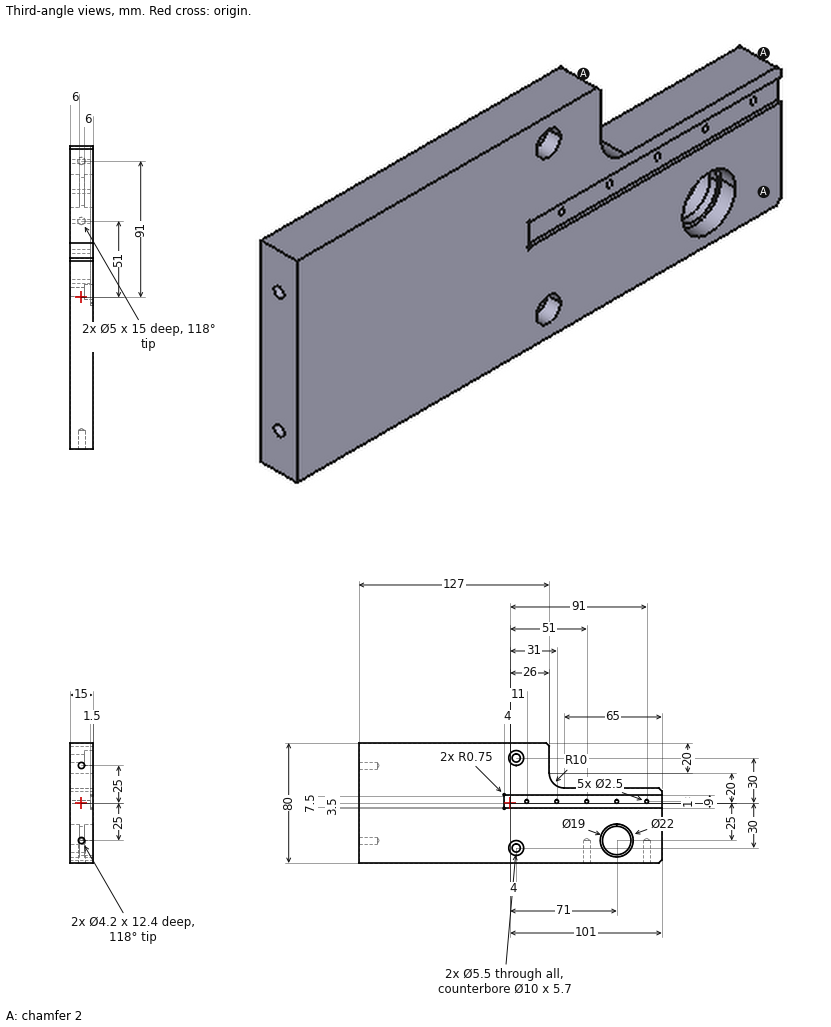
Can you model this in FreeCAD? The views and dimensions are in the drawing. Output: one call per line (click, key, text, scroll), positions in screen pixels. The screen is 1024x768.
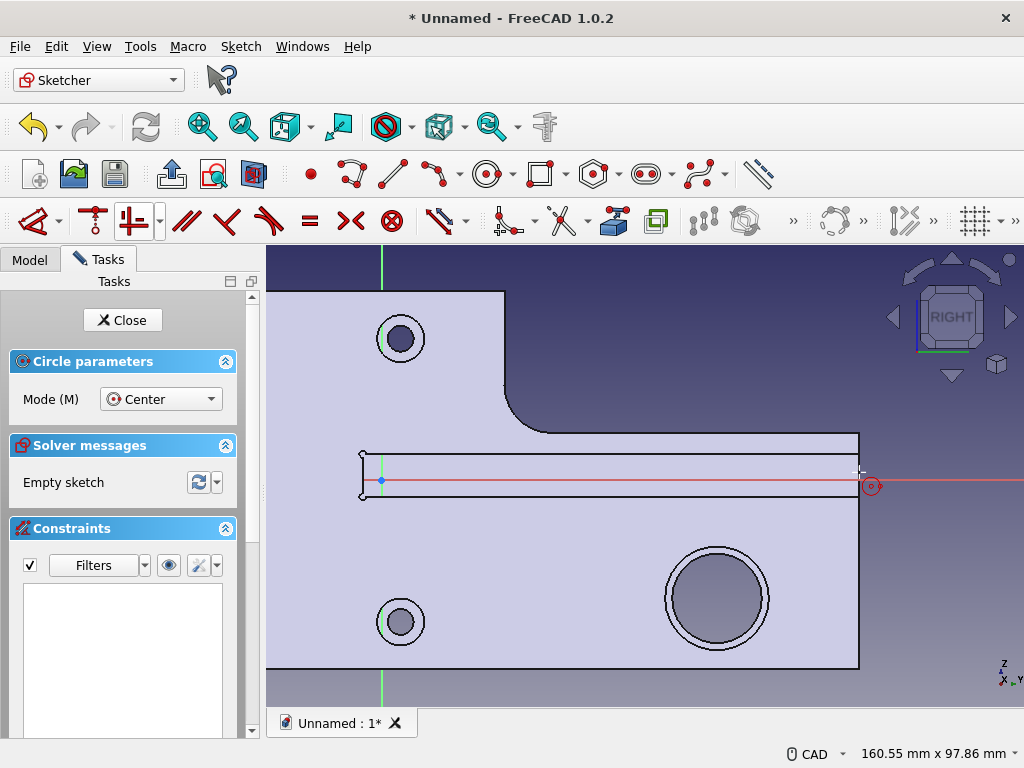
scroll(811, 476, up, 7)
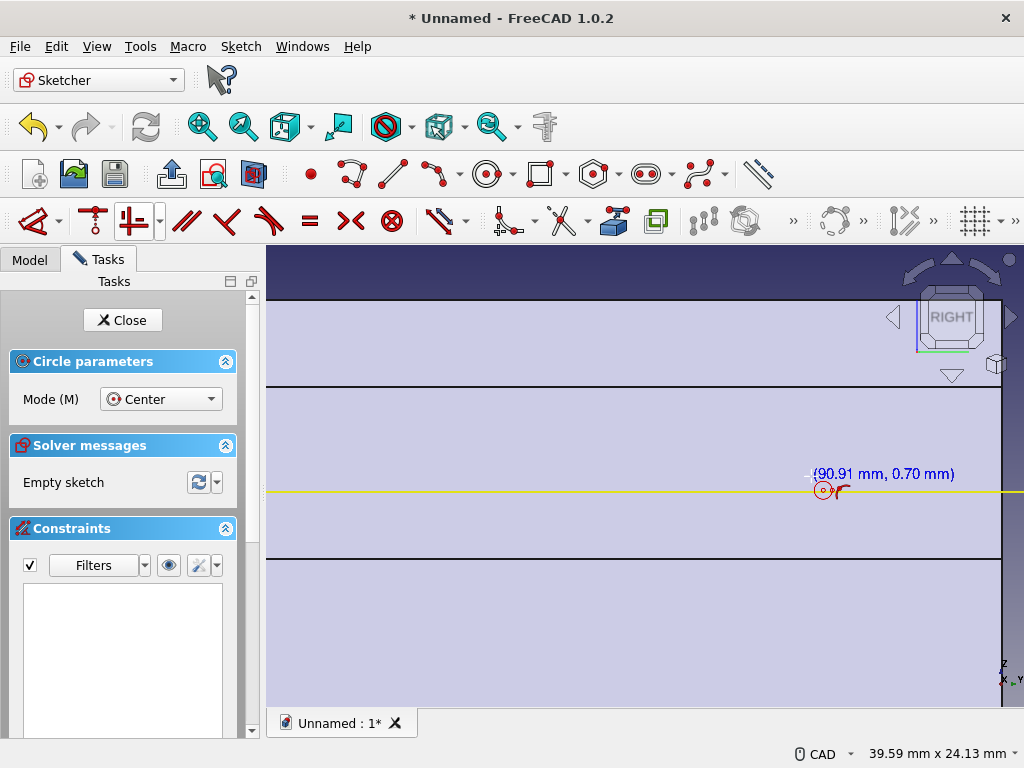
click(810, 473)
click(827, 456)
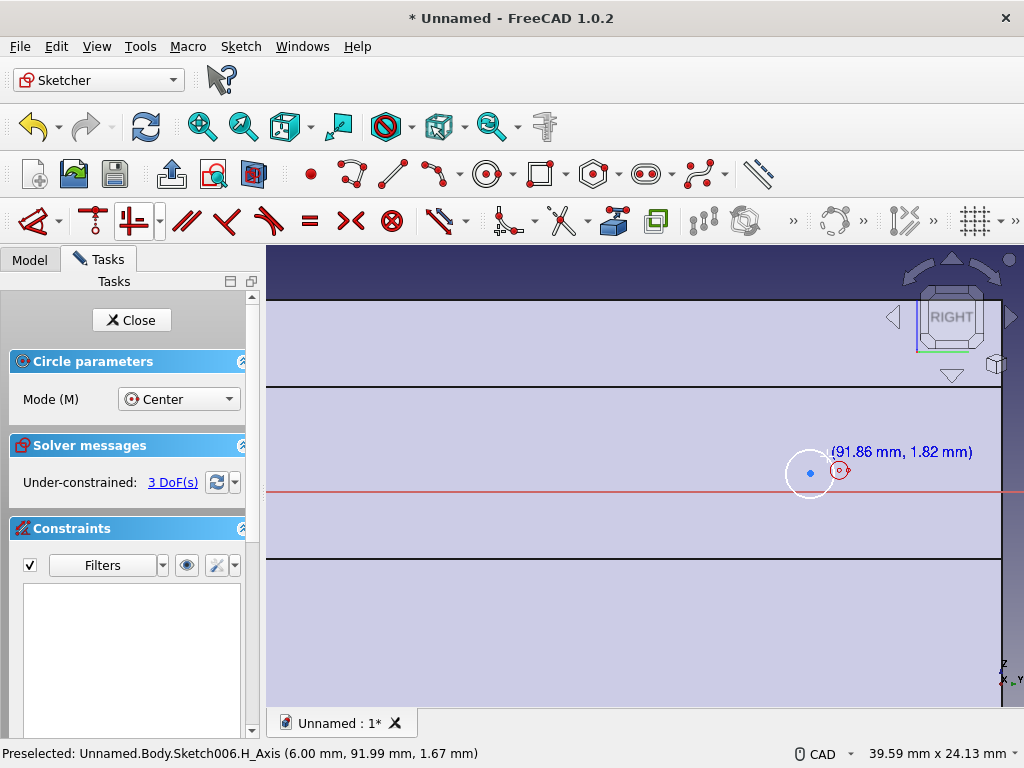
click(428, 473)
click(444, 456)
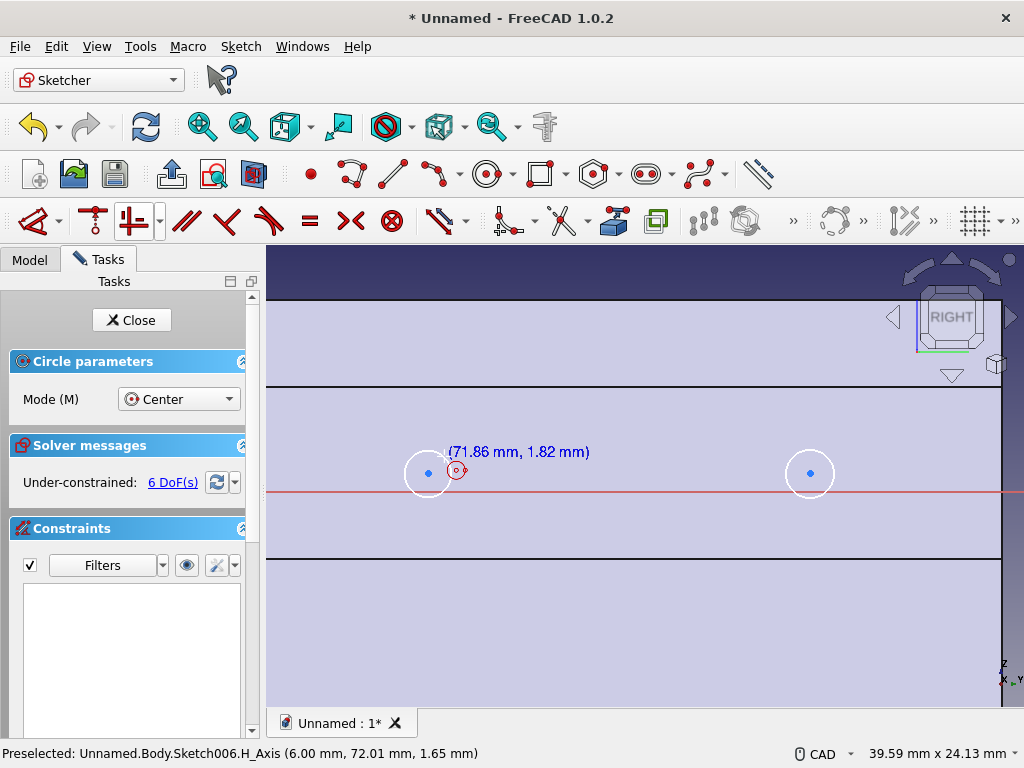
scroll(781, 477, down, 7)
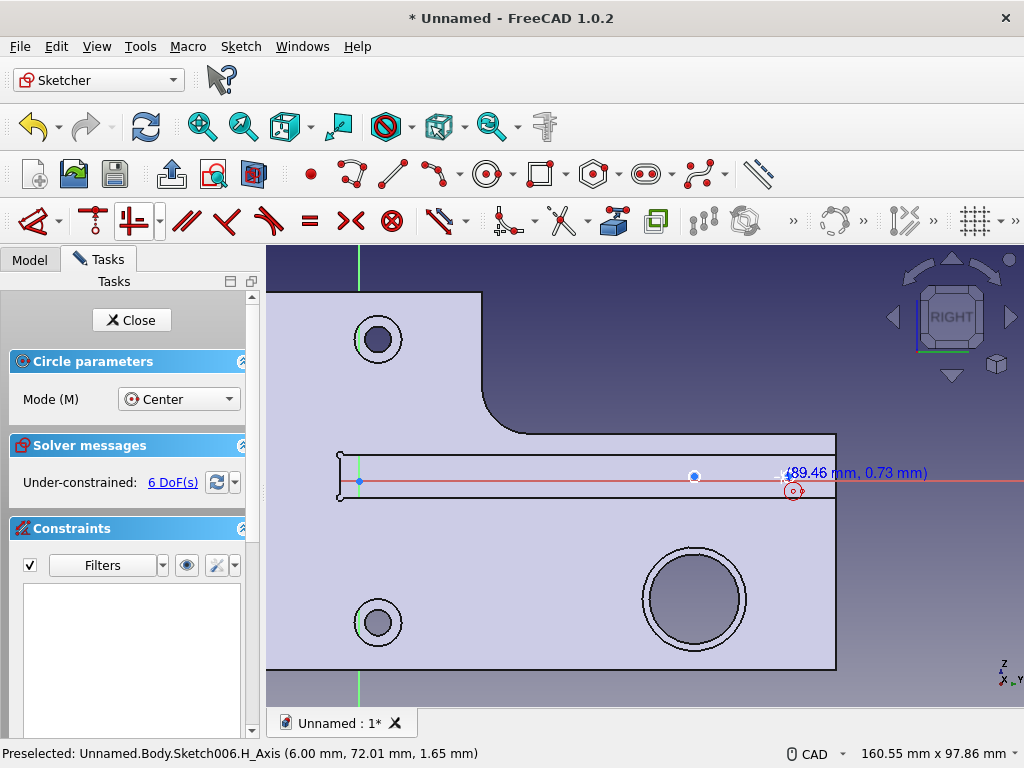
scroll(600, 476, up, 7)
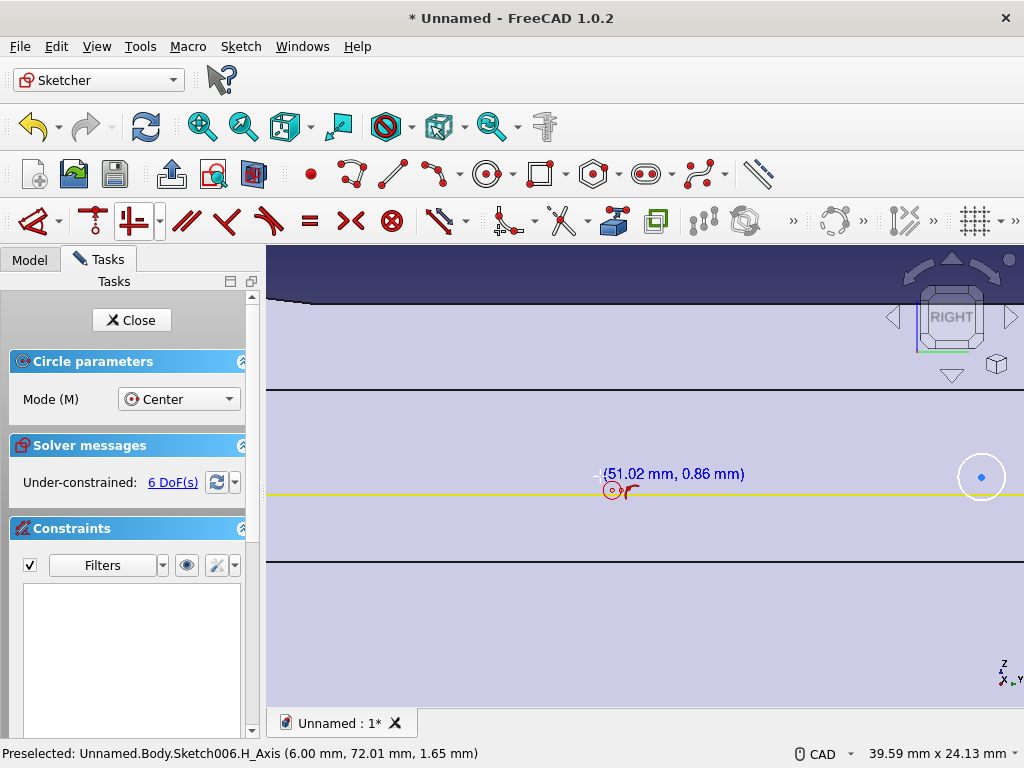
click(598, 476)
click(615, 459)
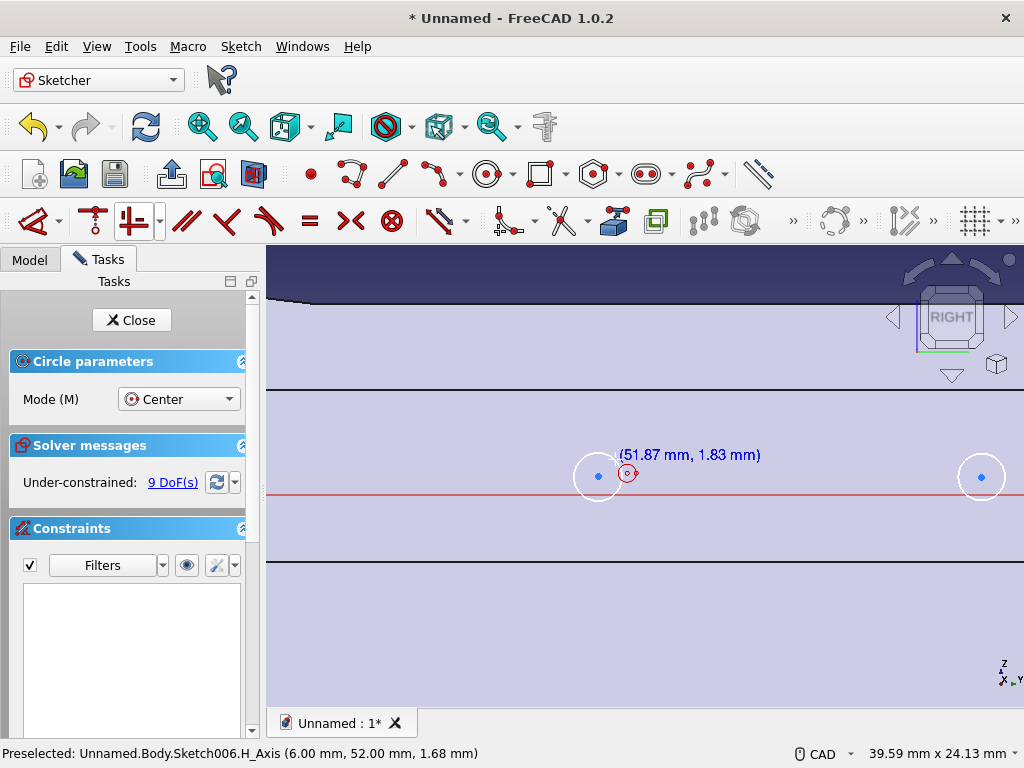
scroll(600, 476, down, 7)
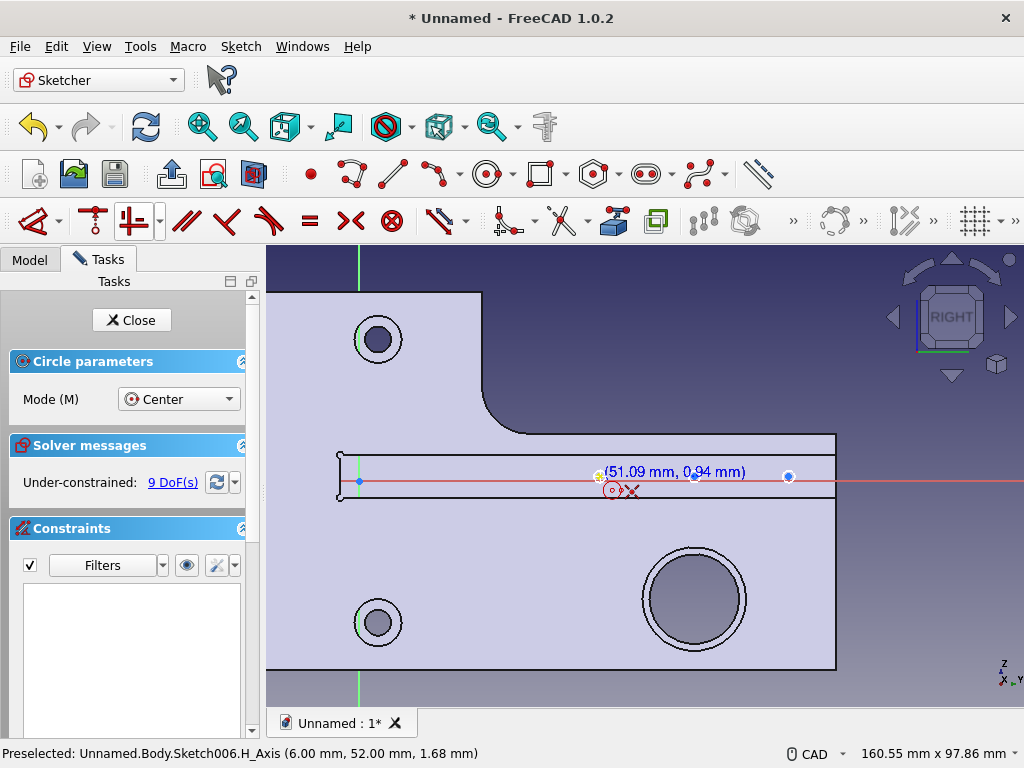
scroll(506, 476, up, 7)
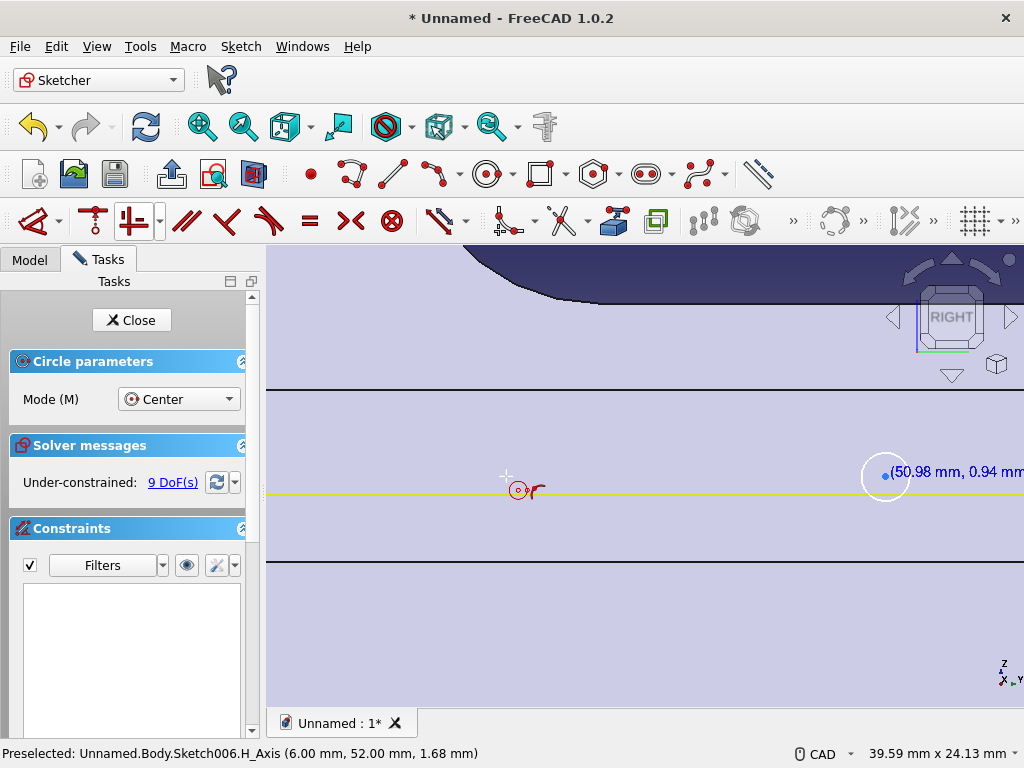
click(503, 476)
click(520, 459)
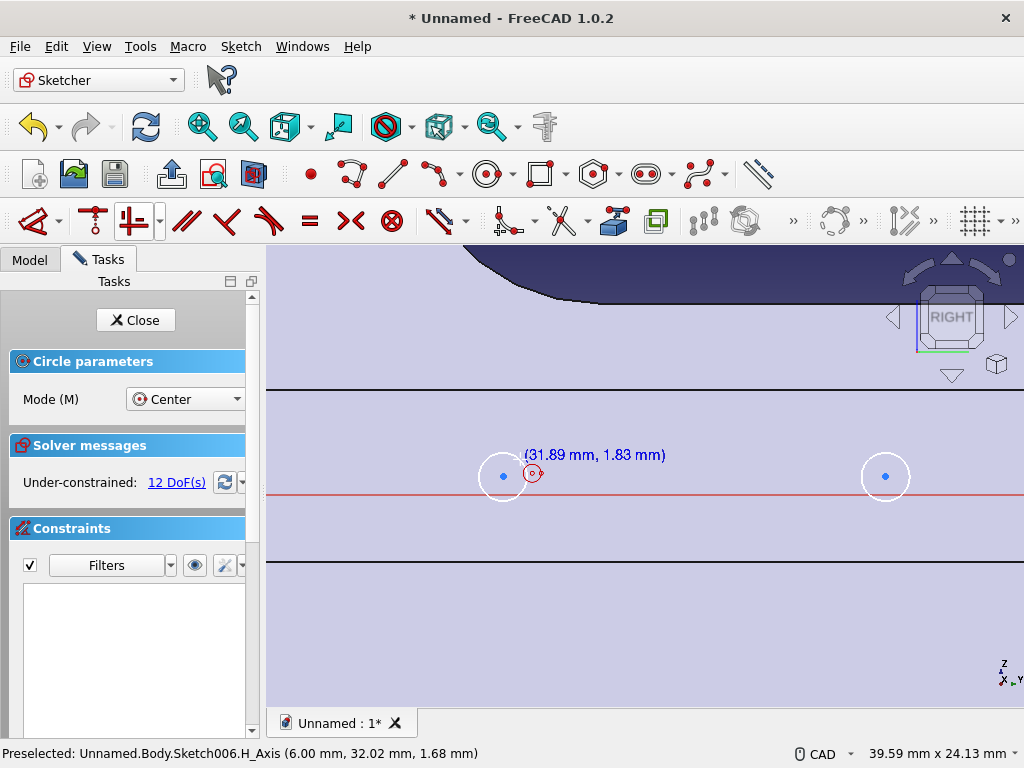
scroll(506, 476, down, 7)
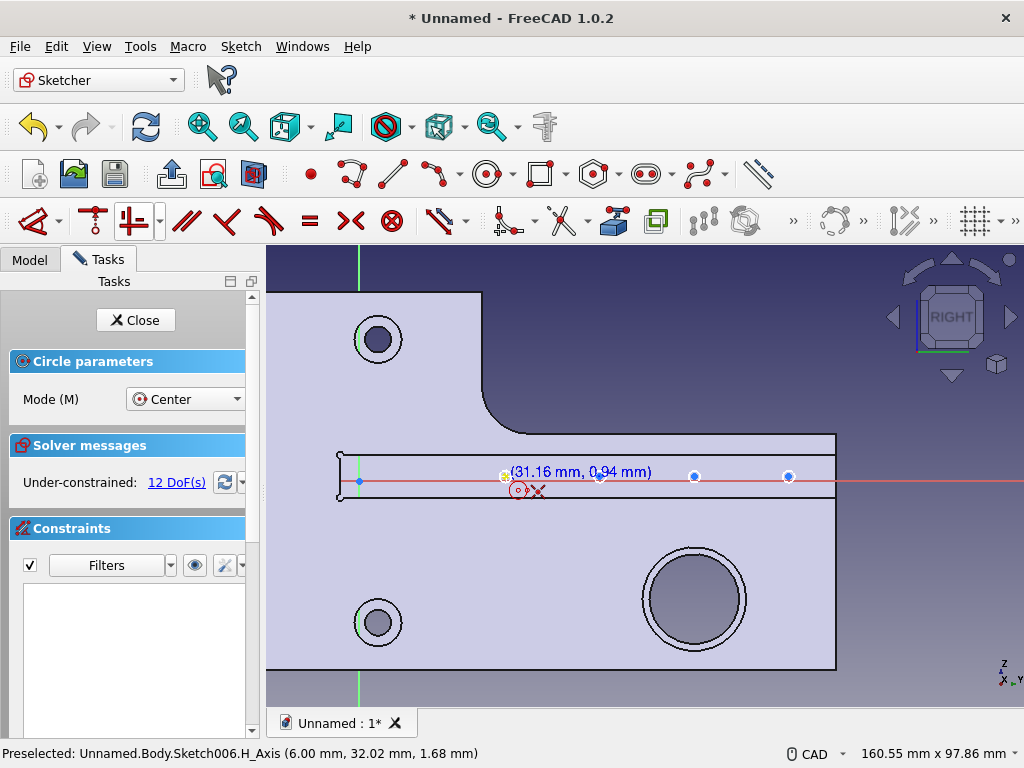
scroll(411, 476, up, 7)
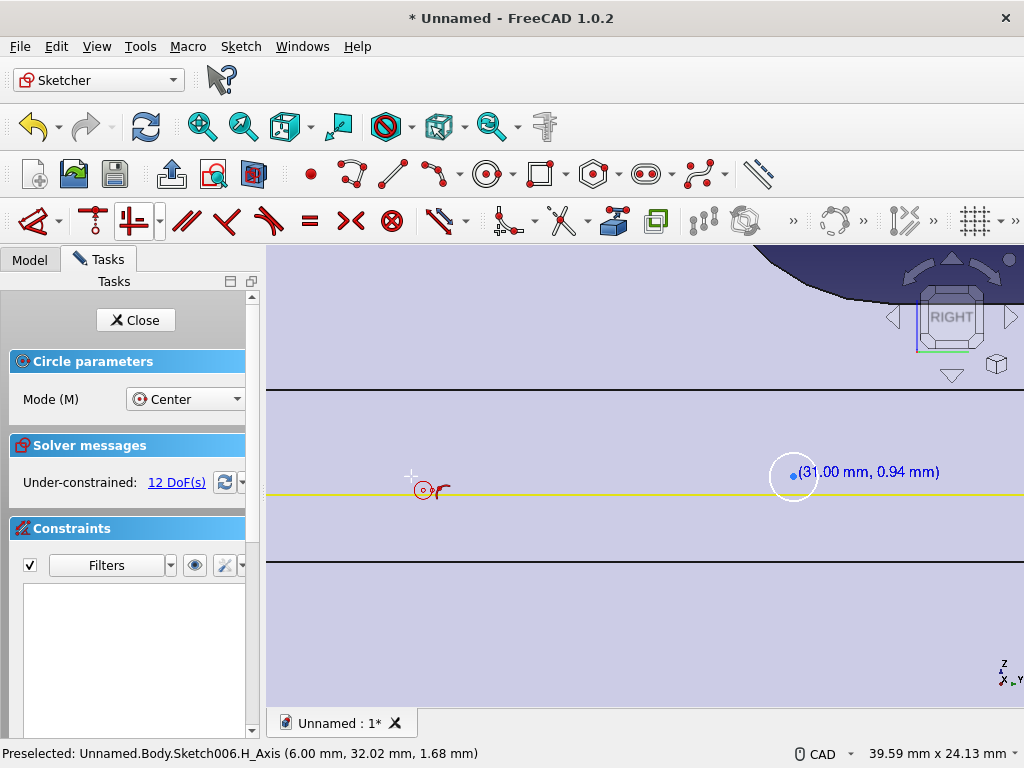
click(411, 476)
click(428, 459)
key(Escape)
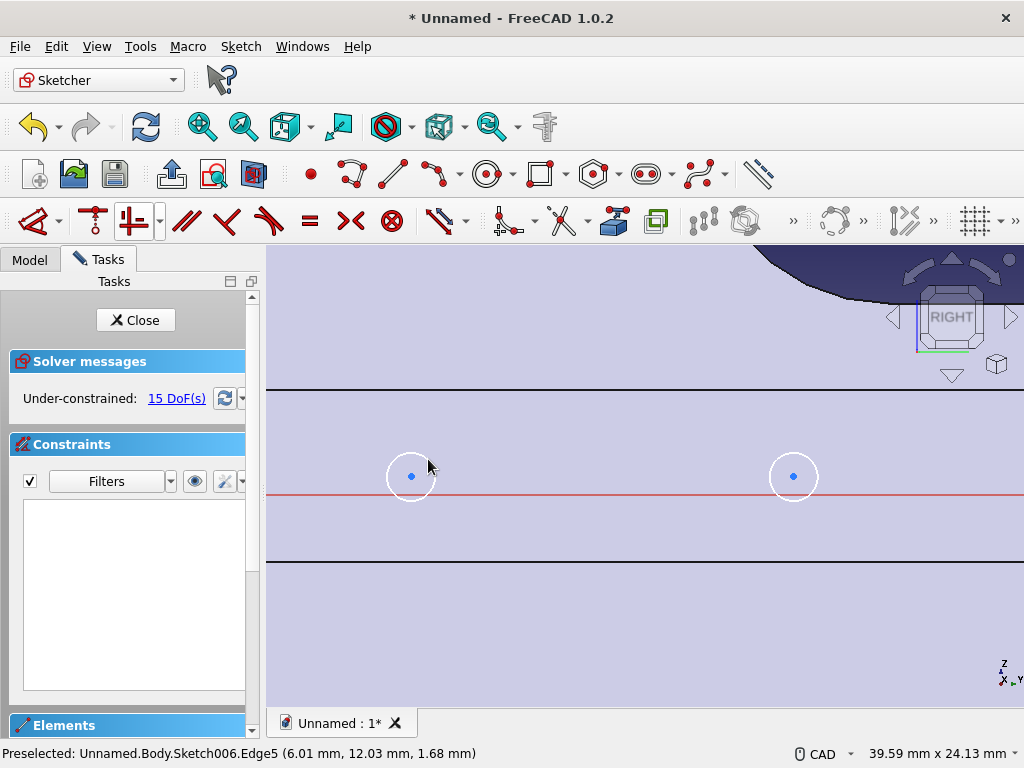
scroll(411, 476, down, 7)